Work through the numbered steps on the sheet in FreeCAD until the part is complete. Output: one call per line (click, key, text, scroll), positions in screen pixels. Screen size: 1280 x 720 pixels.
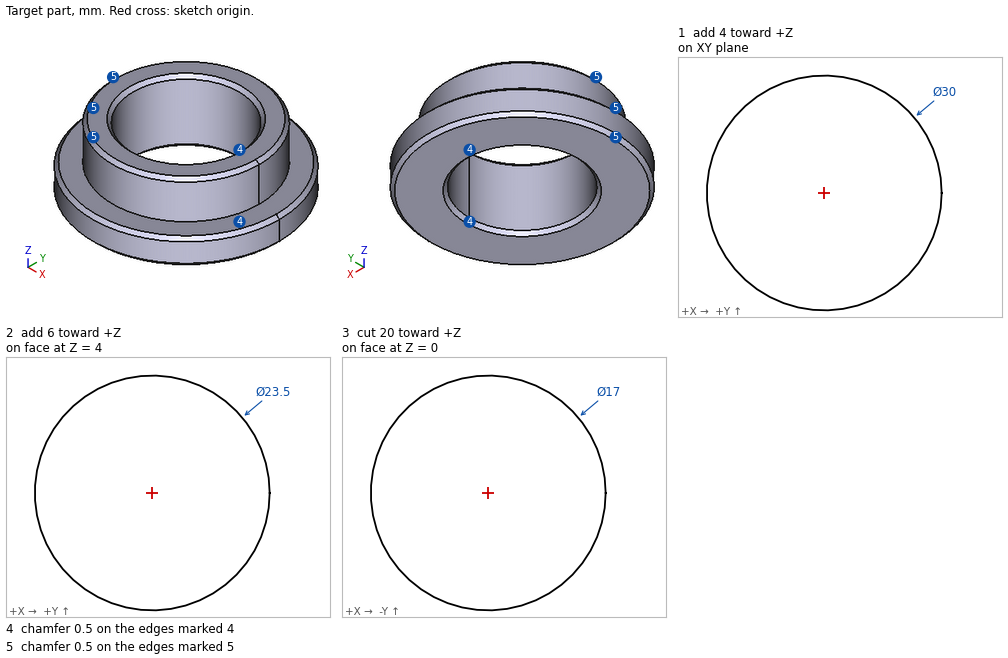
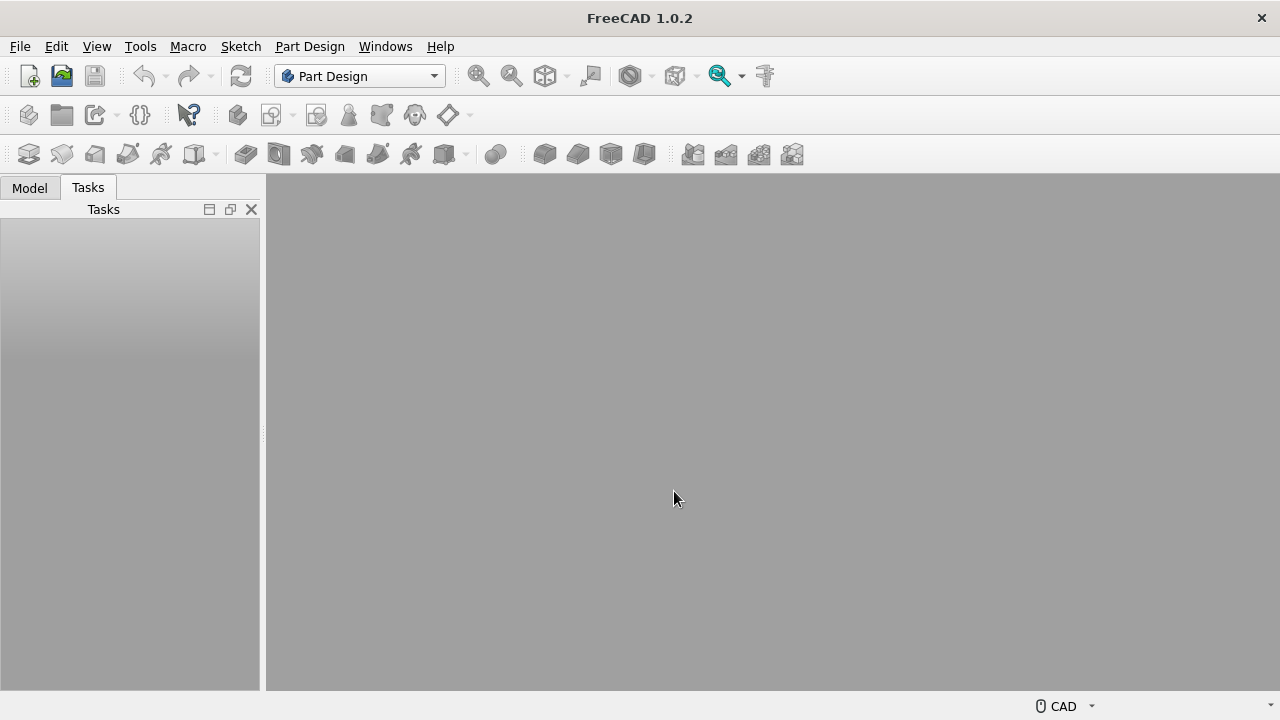
click(29, 76)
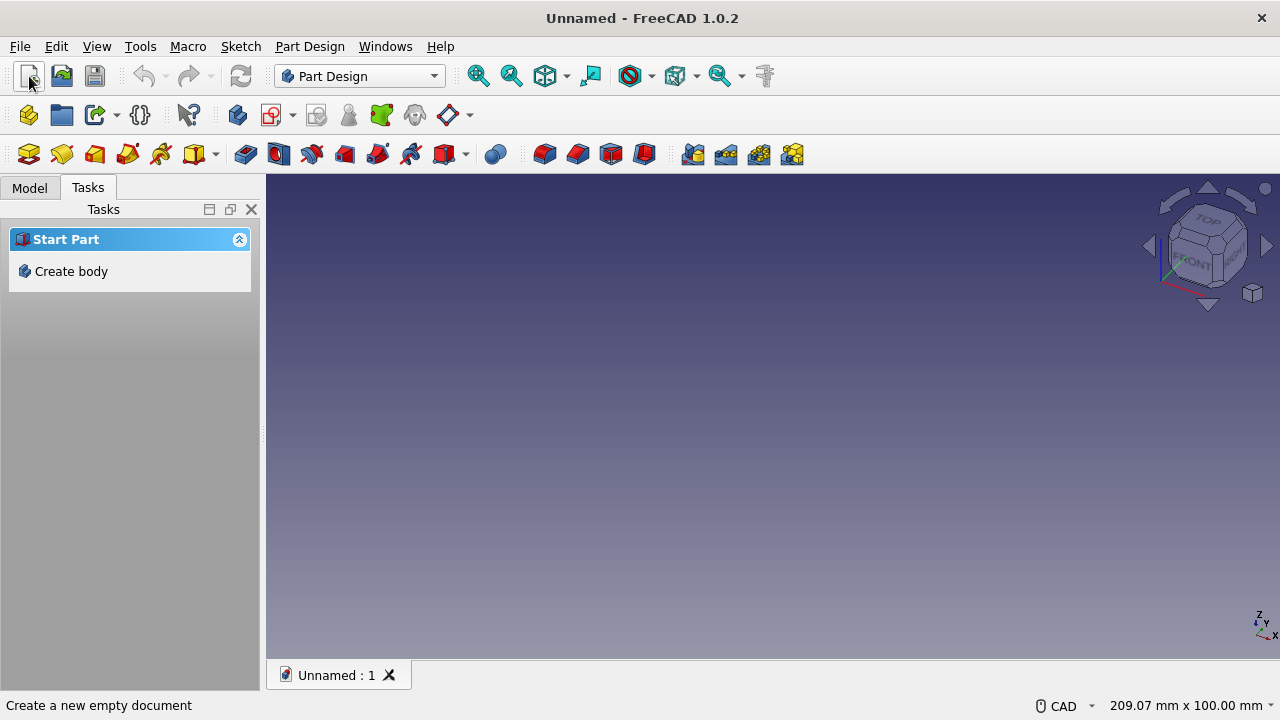
click(270, 116)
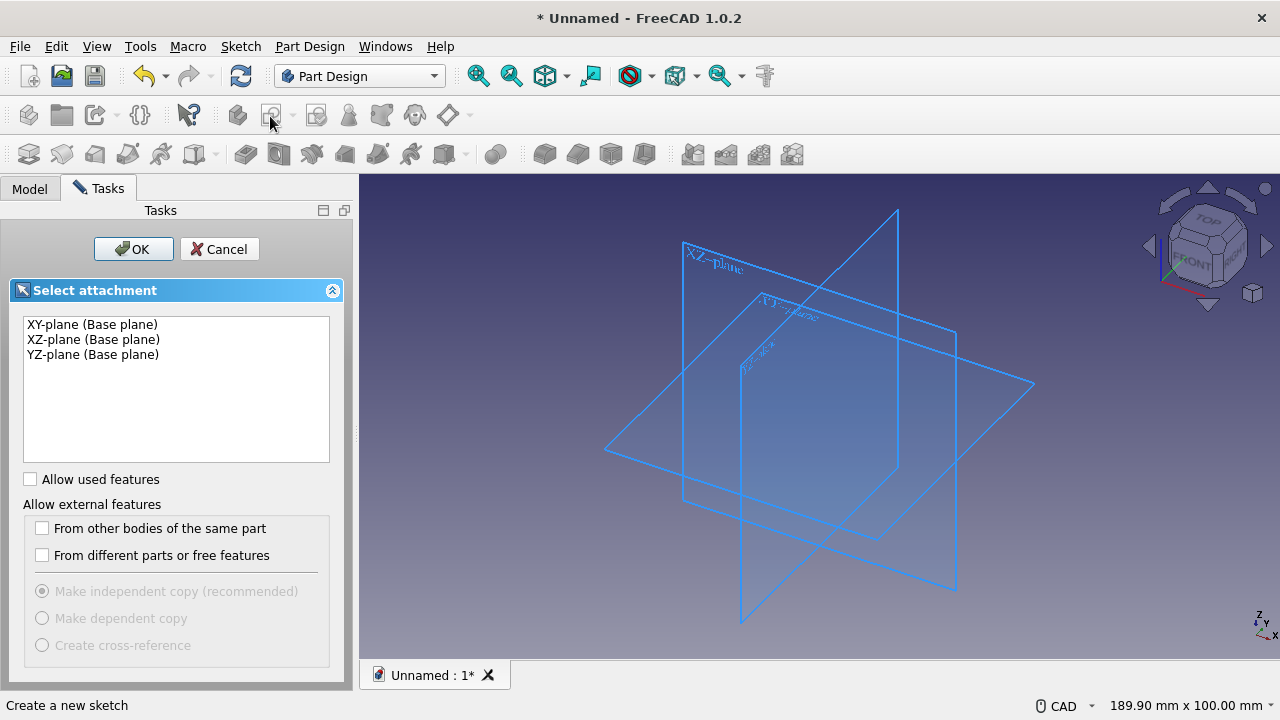
click(84, 324)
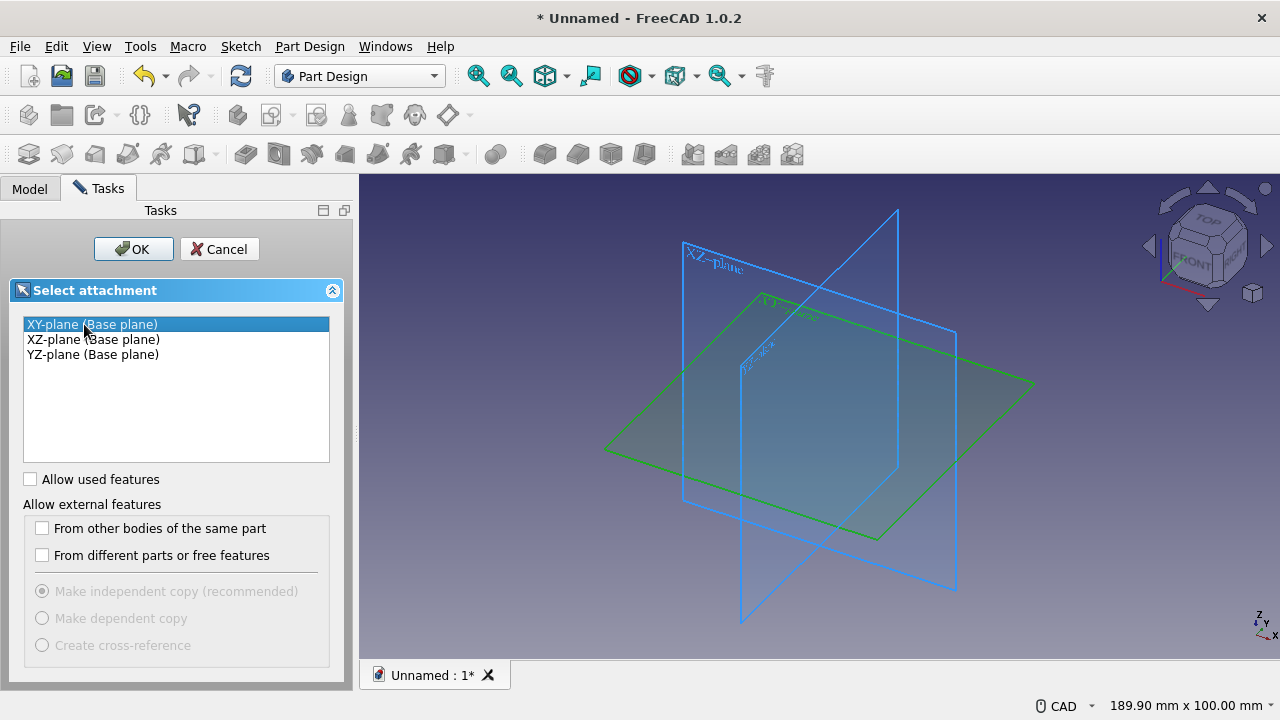
click(134, 249)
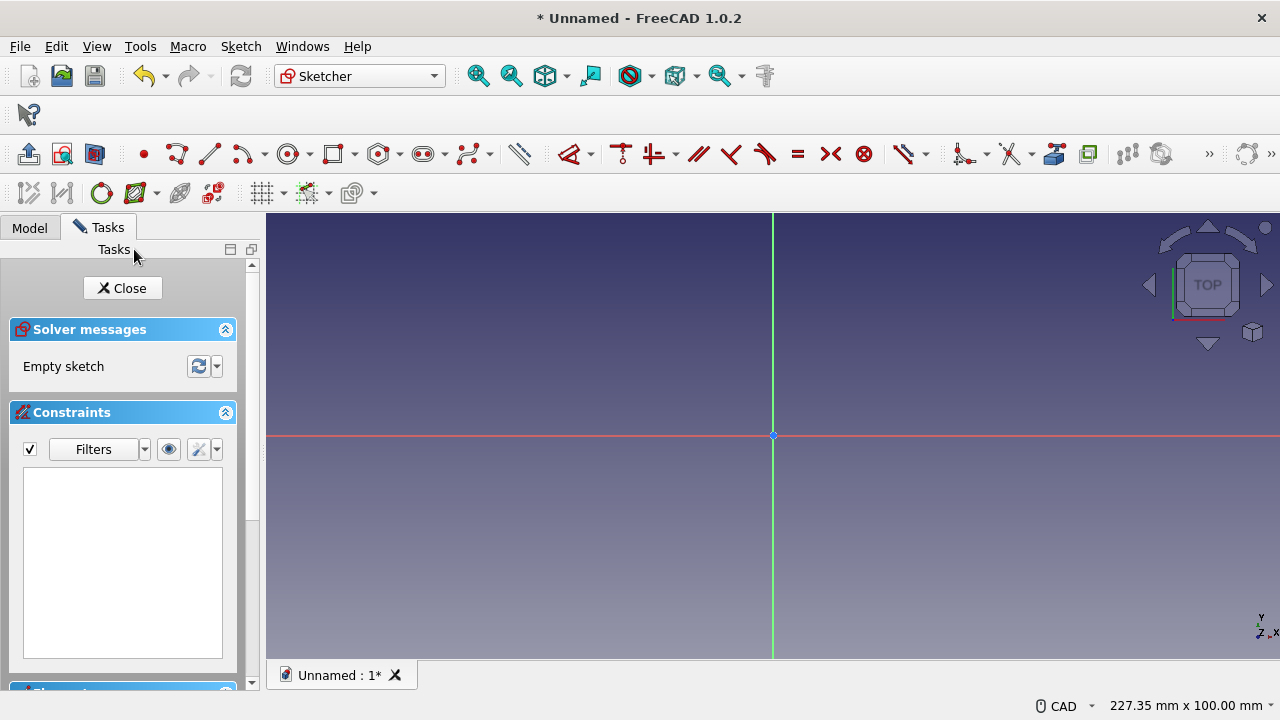
scroll(829, 436, up, 4)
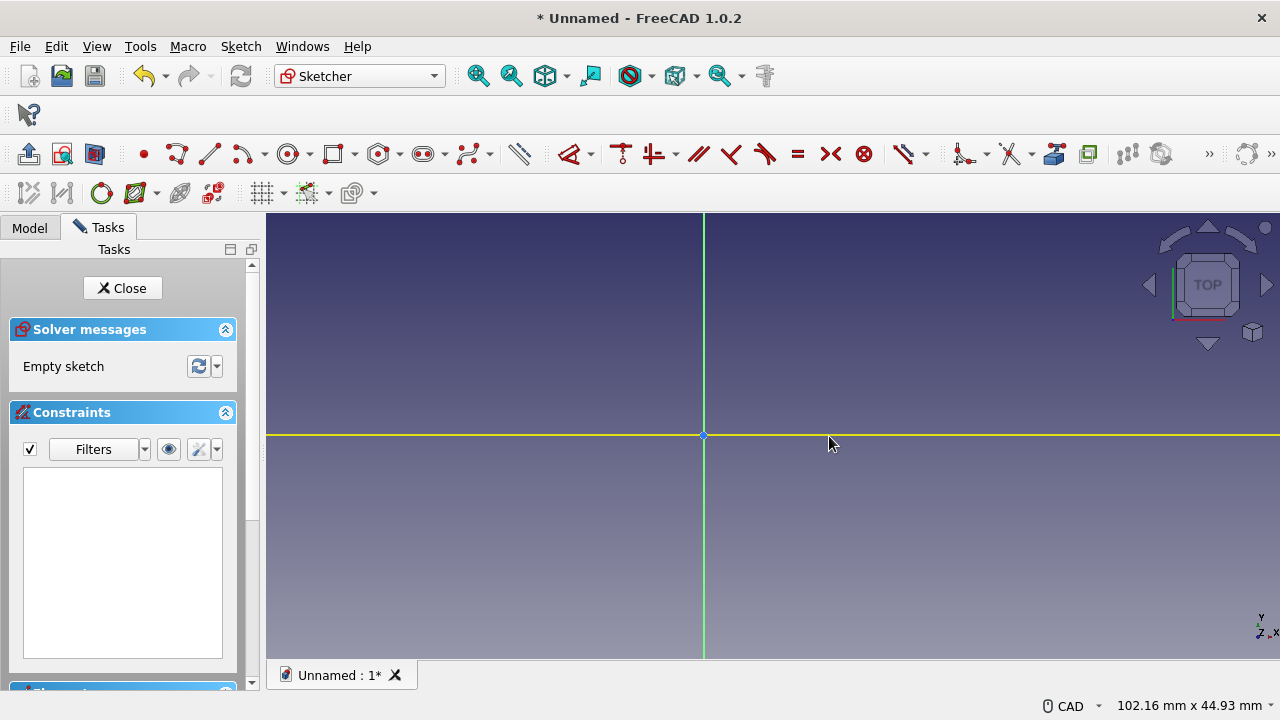
click(288, 154)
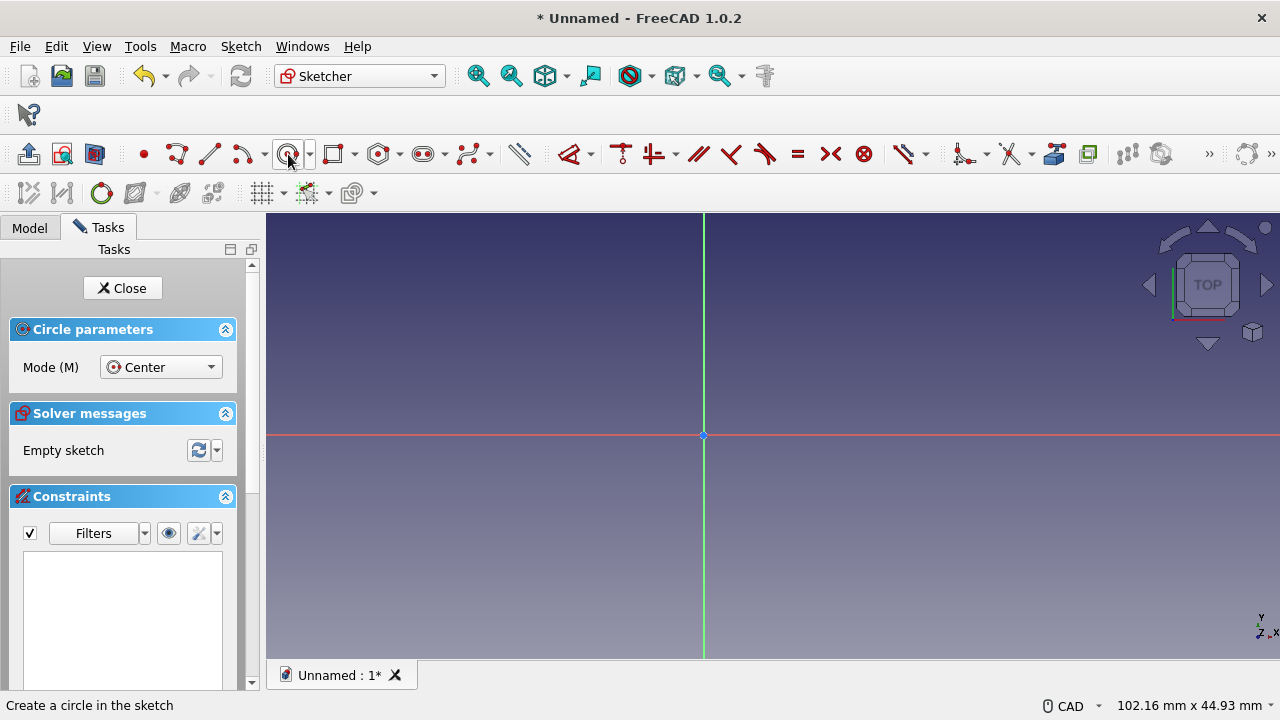
click(704, 435)
move(809, 330)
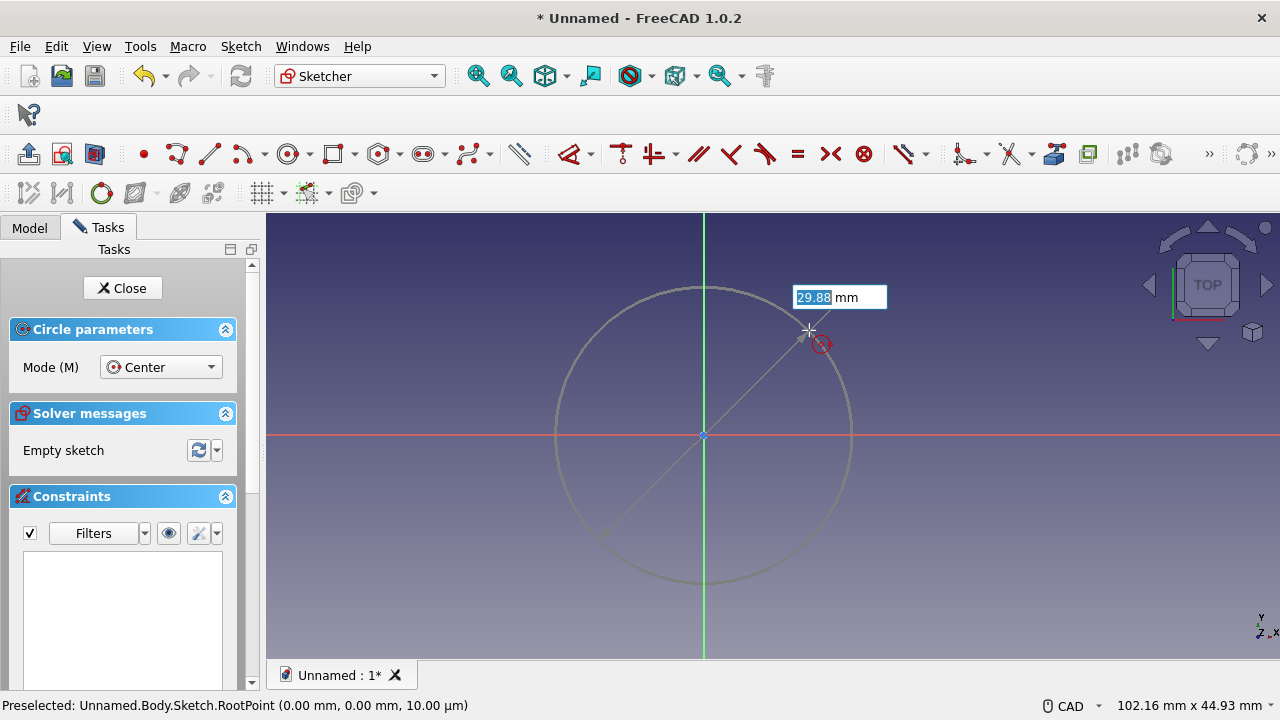
text(30)
key(Return)
key(Escape)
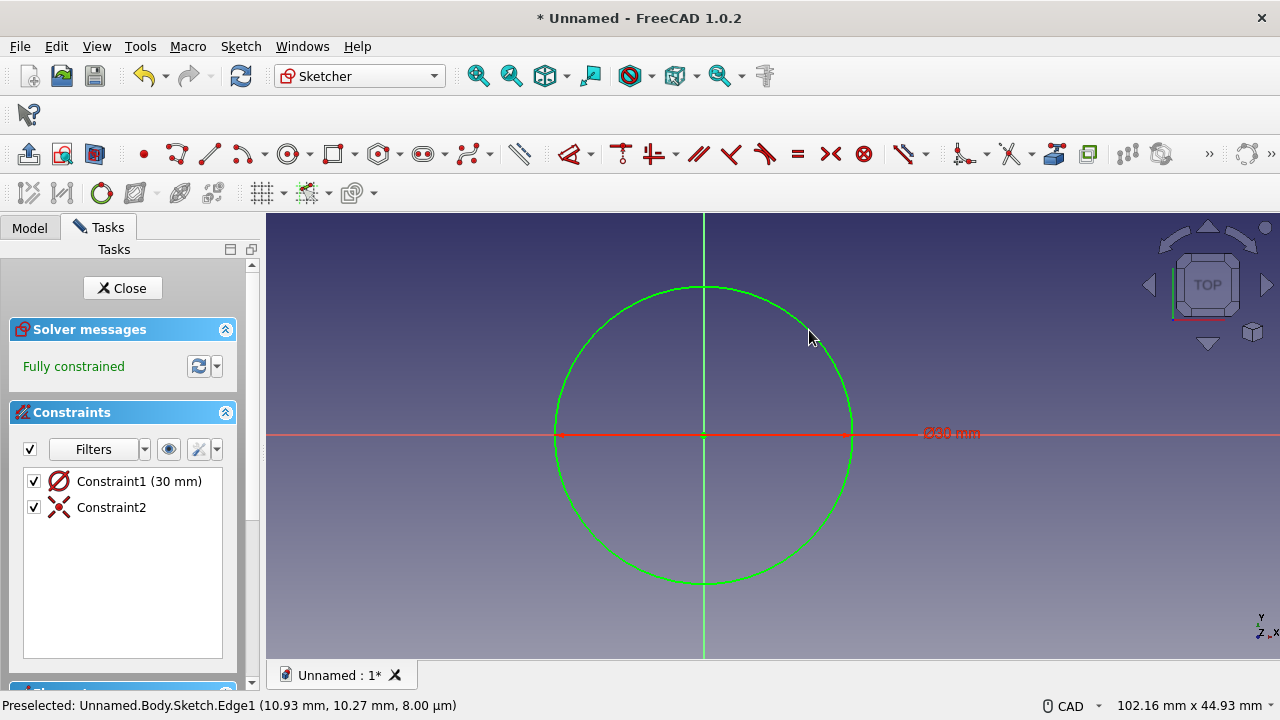
click(123, 288)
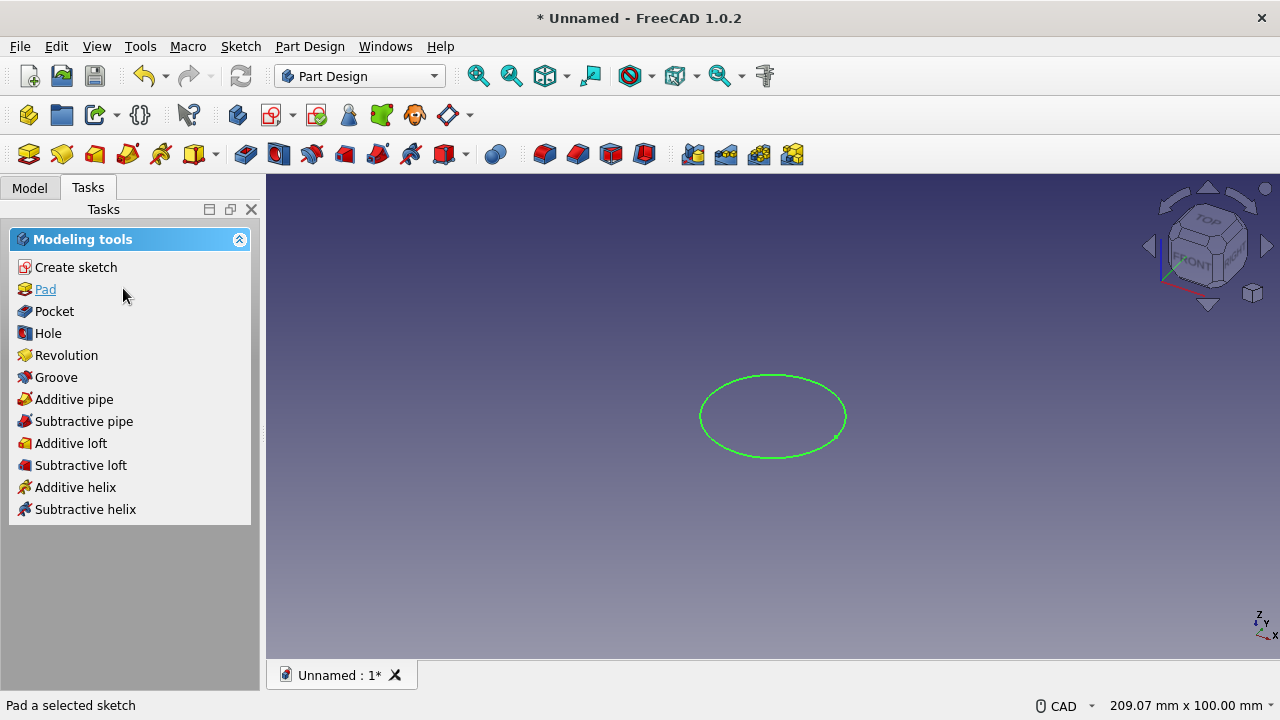
click(29, 154)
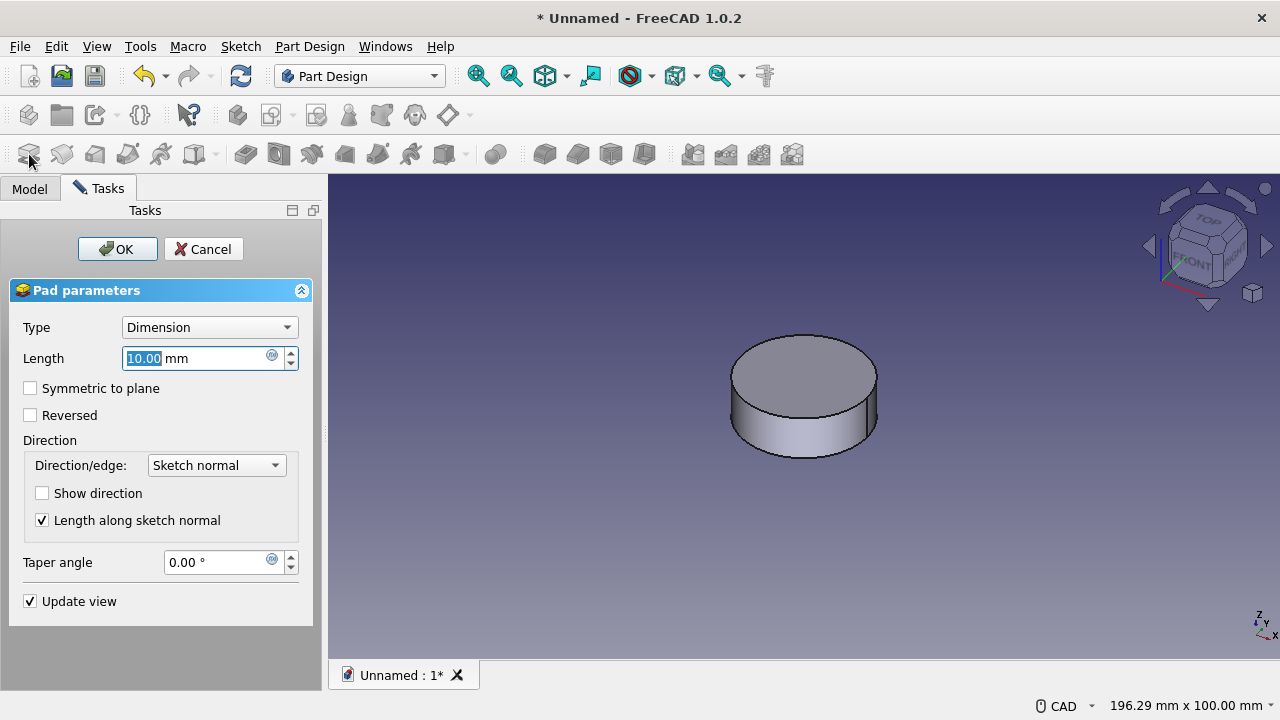
text(4)
key(Tab)